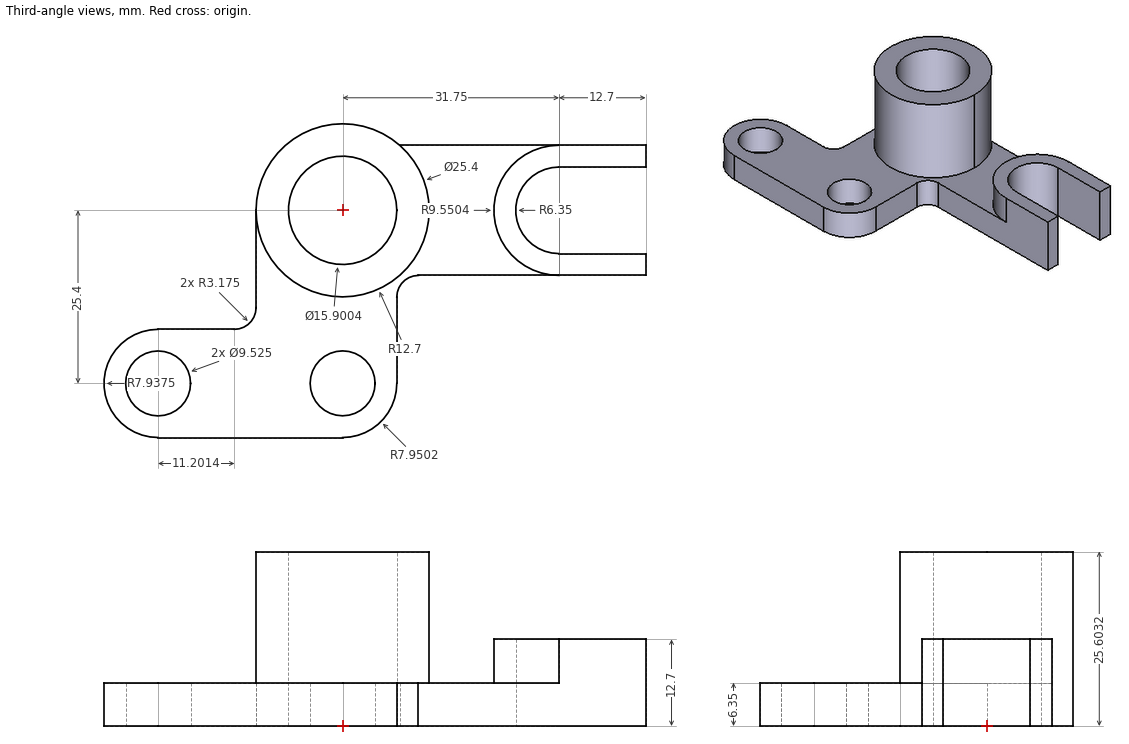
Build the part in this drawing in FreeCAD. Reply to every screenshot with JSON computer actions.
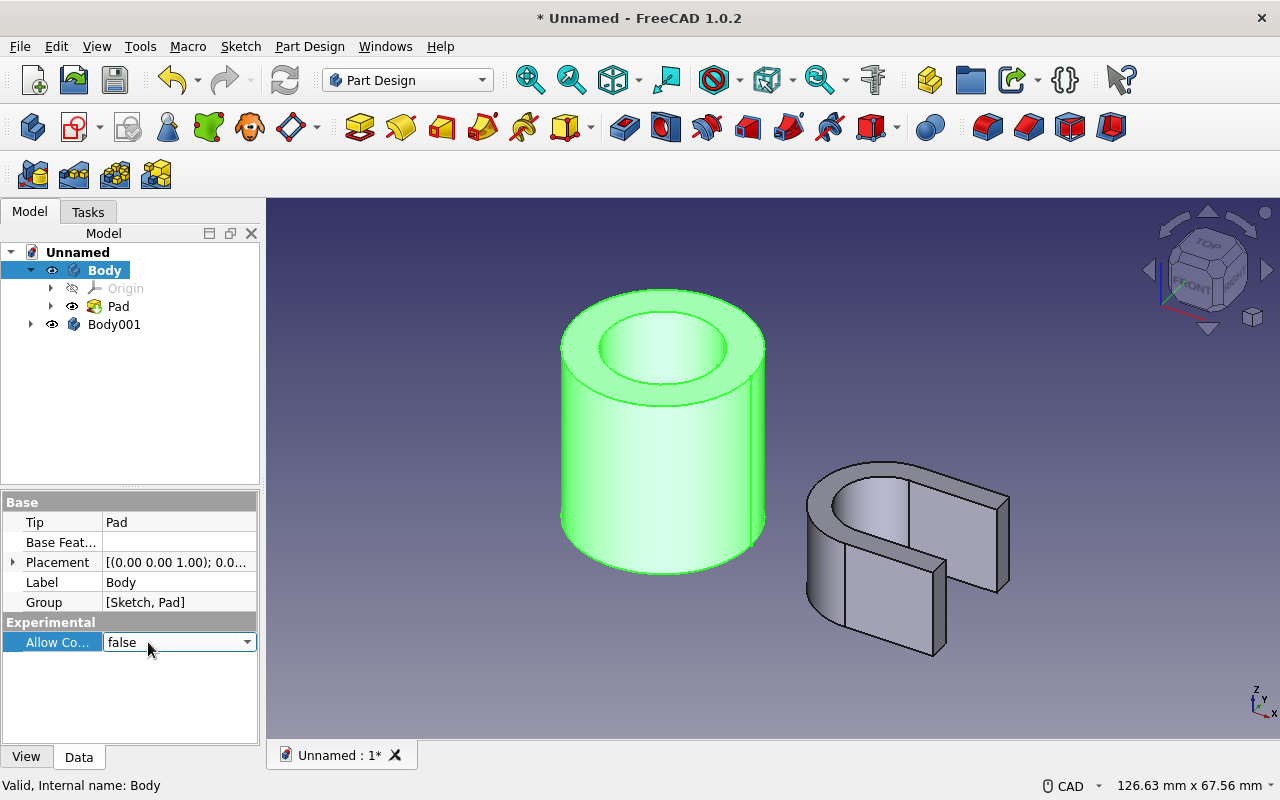
{"action": "left_click", "coordinate": [148, 642]}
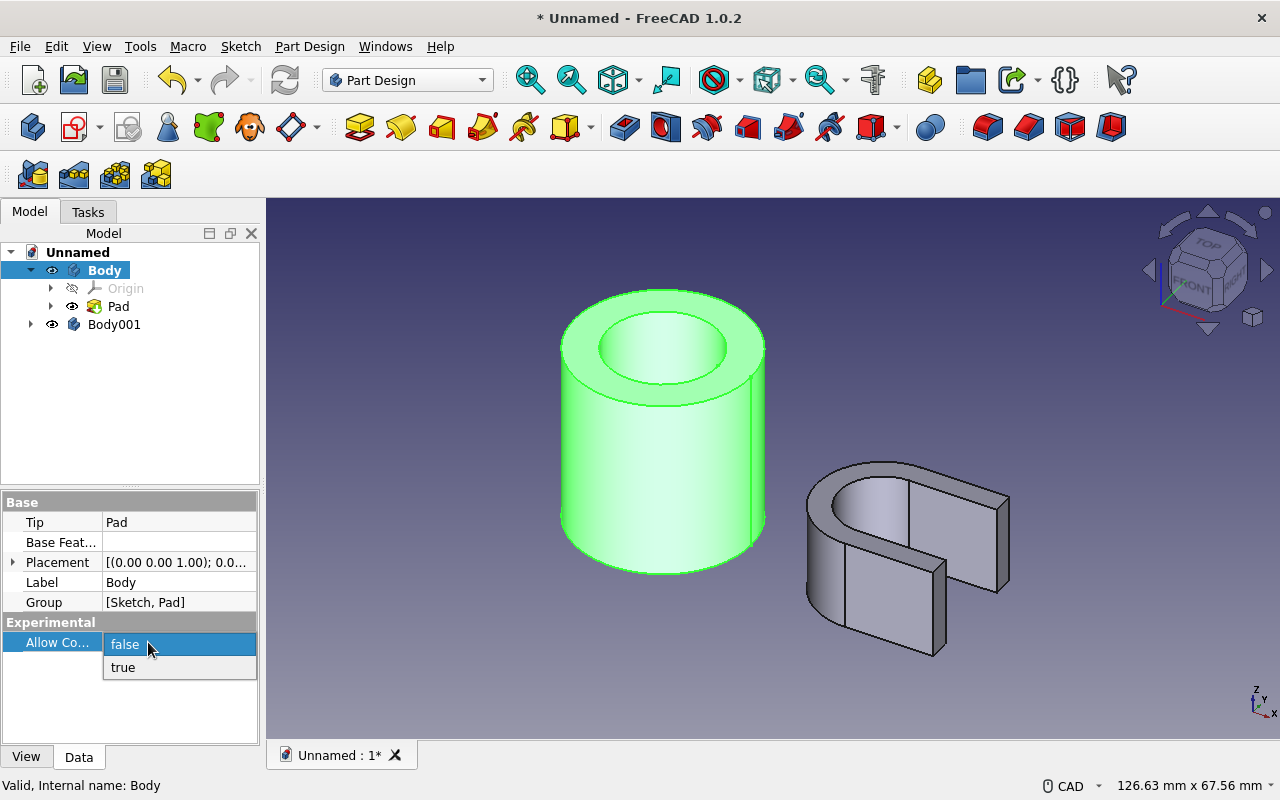
{"action": "left_click", "coordinate": [178, 668]}
{"action": "key", "text": "Return"}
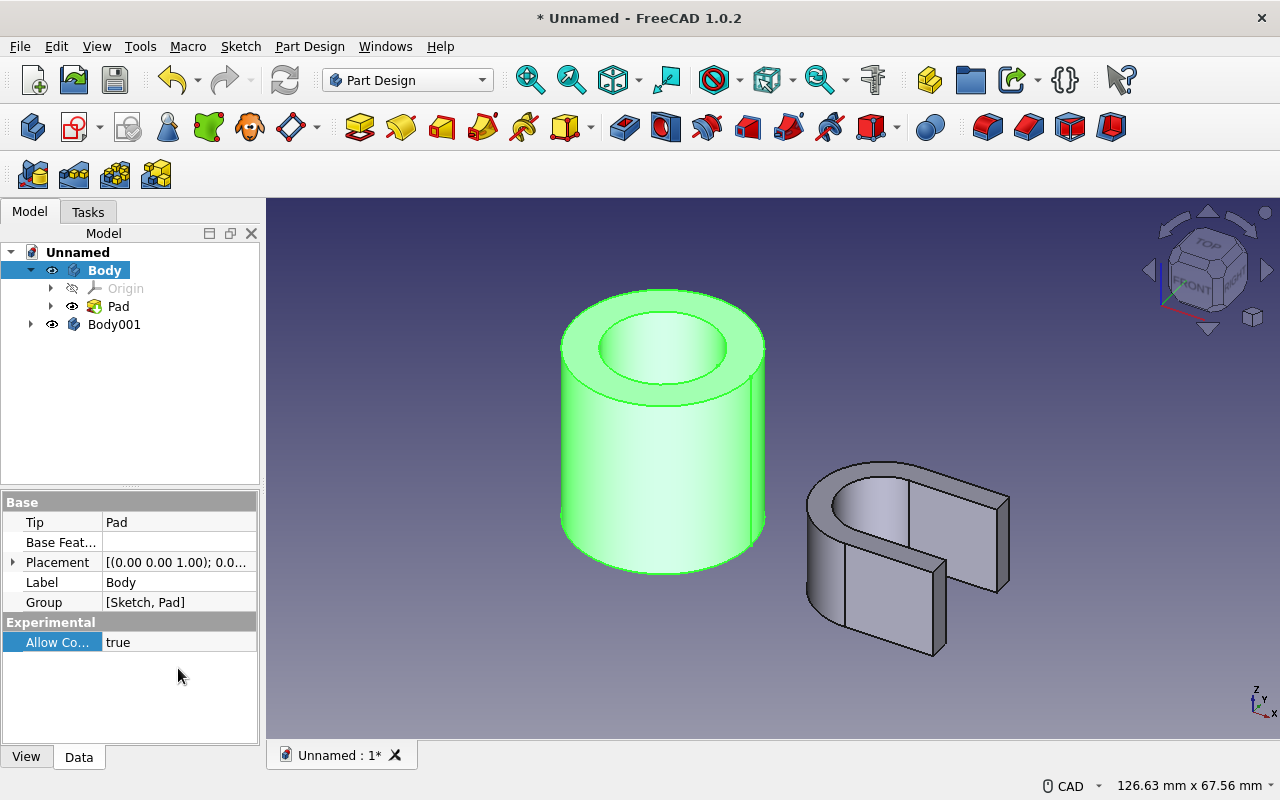
{"action": "left_click", "coordinate": [97, 324]}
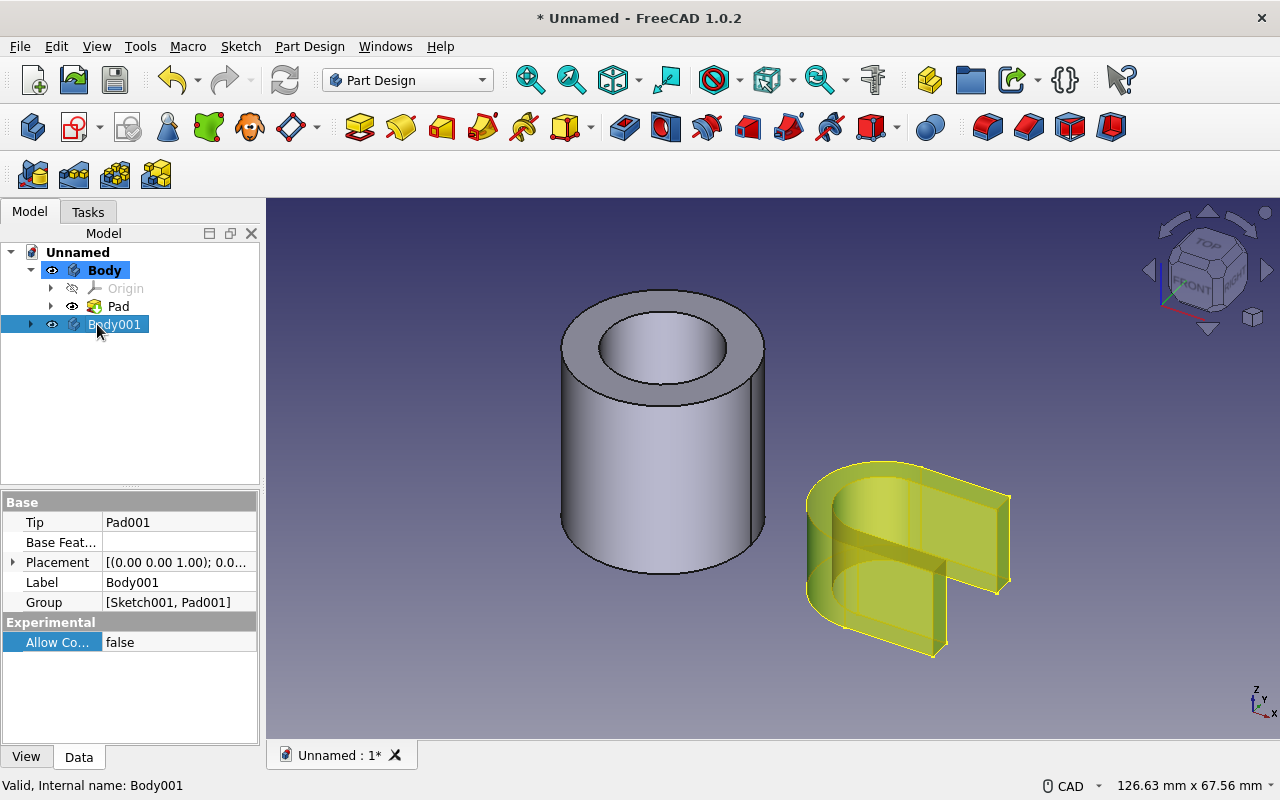
{"action": "left_click", "coordinate": [931, 128]}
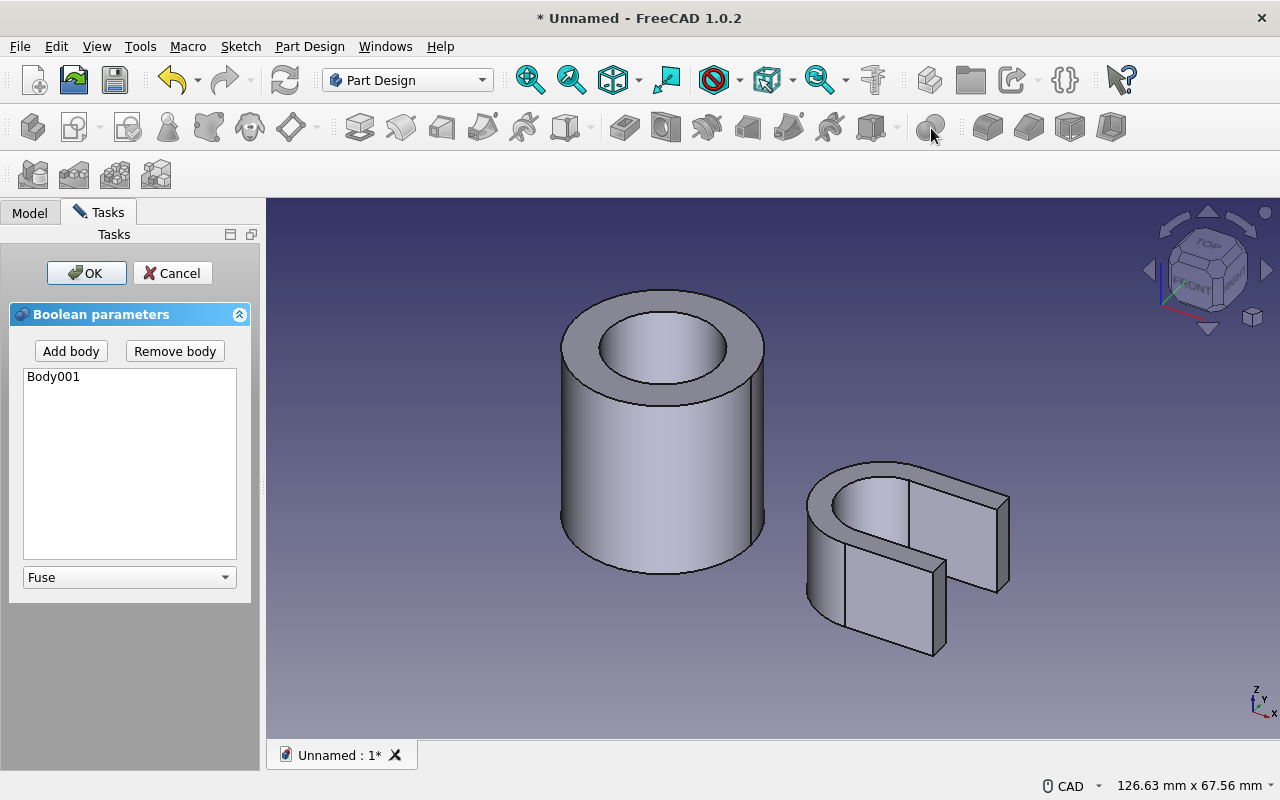
{"action": "left_click", "coordinate": [87, 273]}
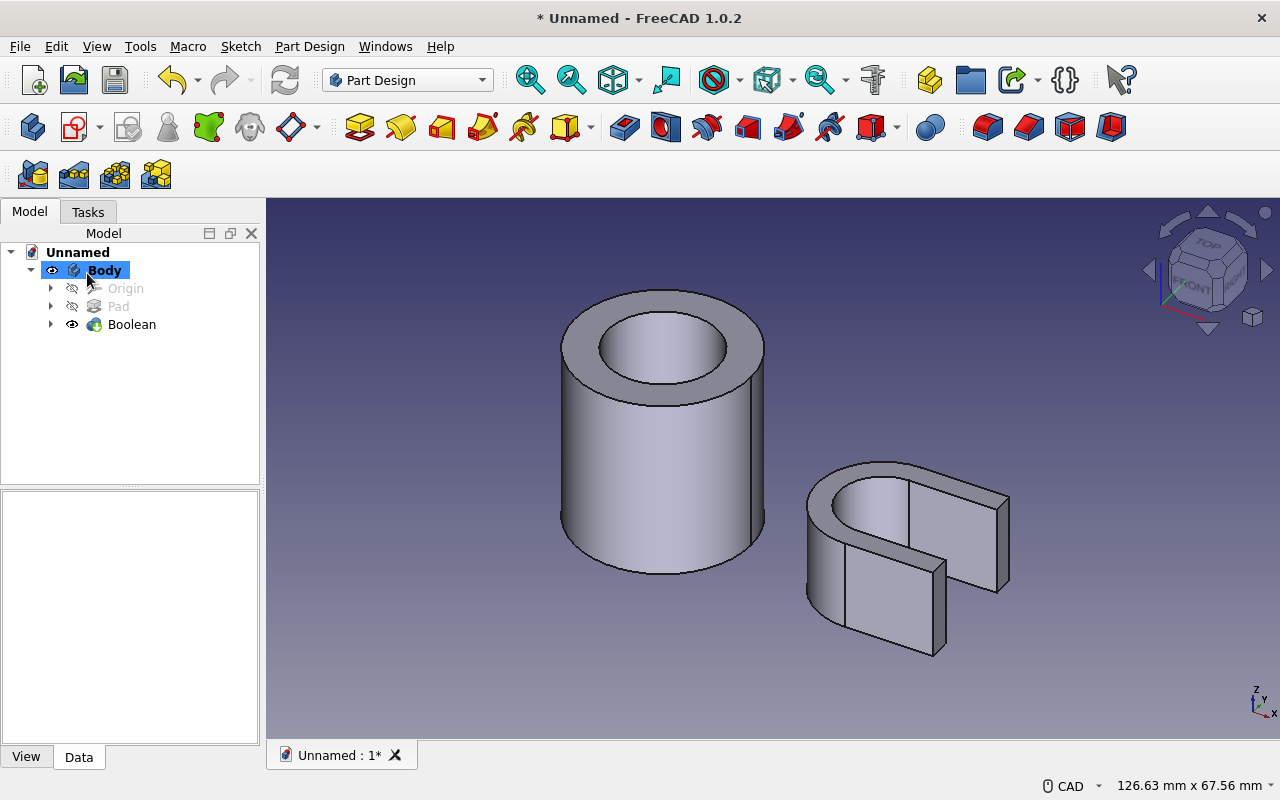
{"action": "left_click", "coordinate": [74, 128]}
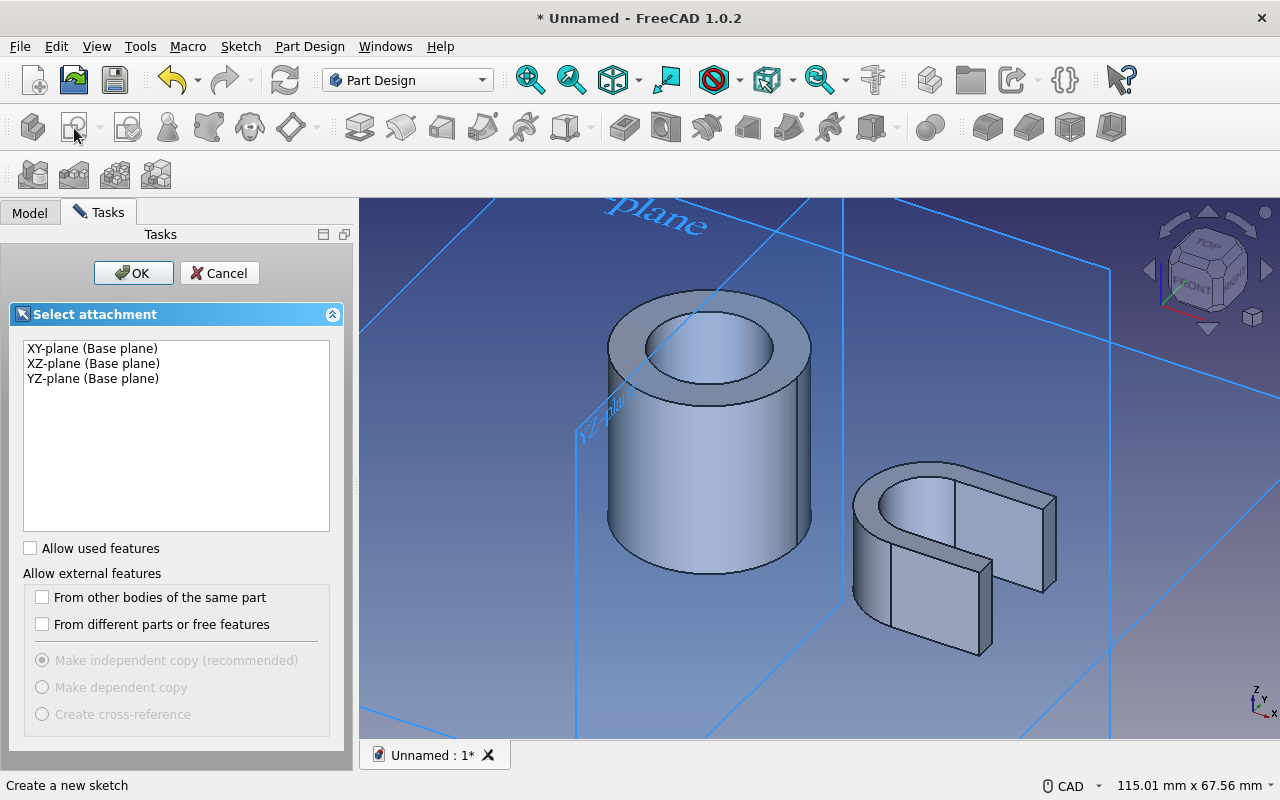
{"action": "left_click", "coordinate": [84, 348]}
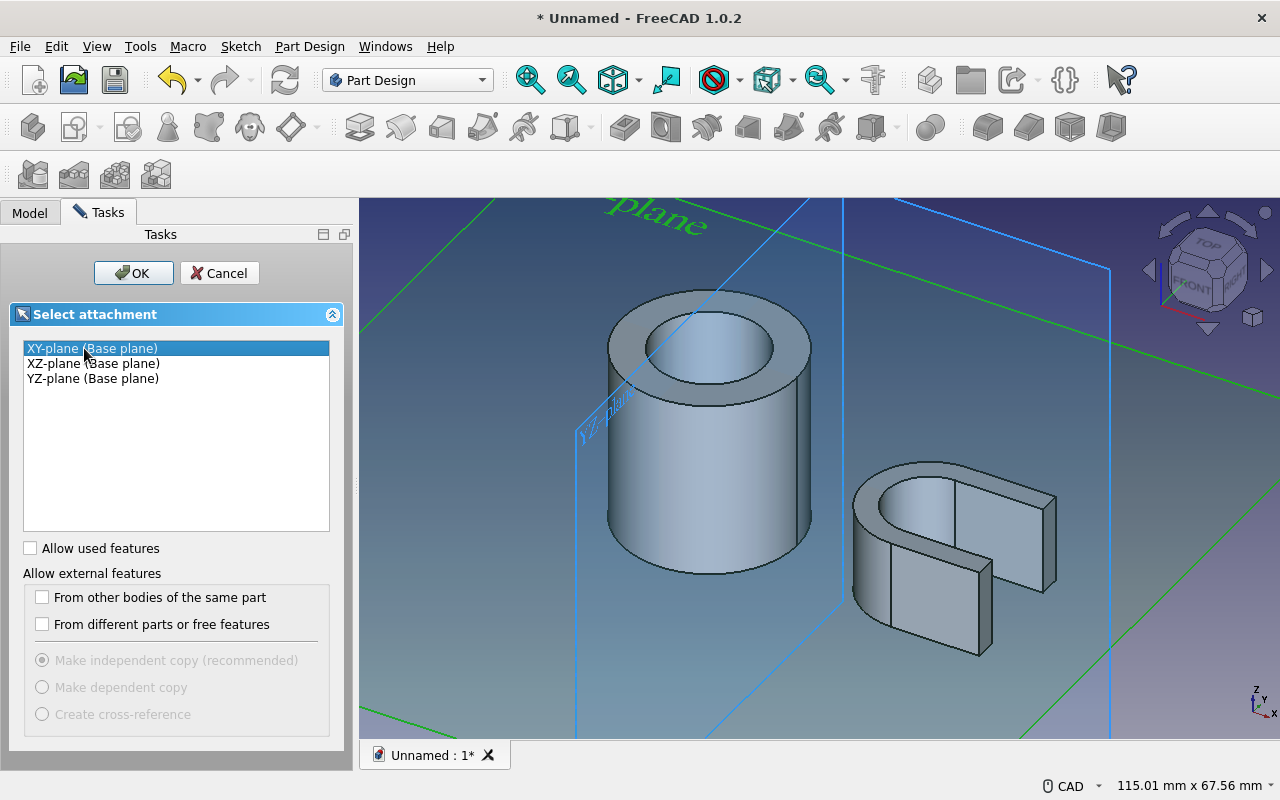
{"action": "left_click", "coordinate": [134, 273]}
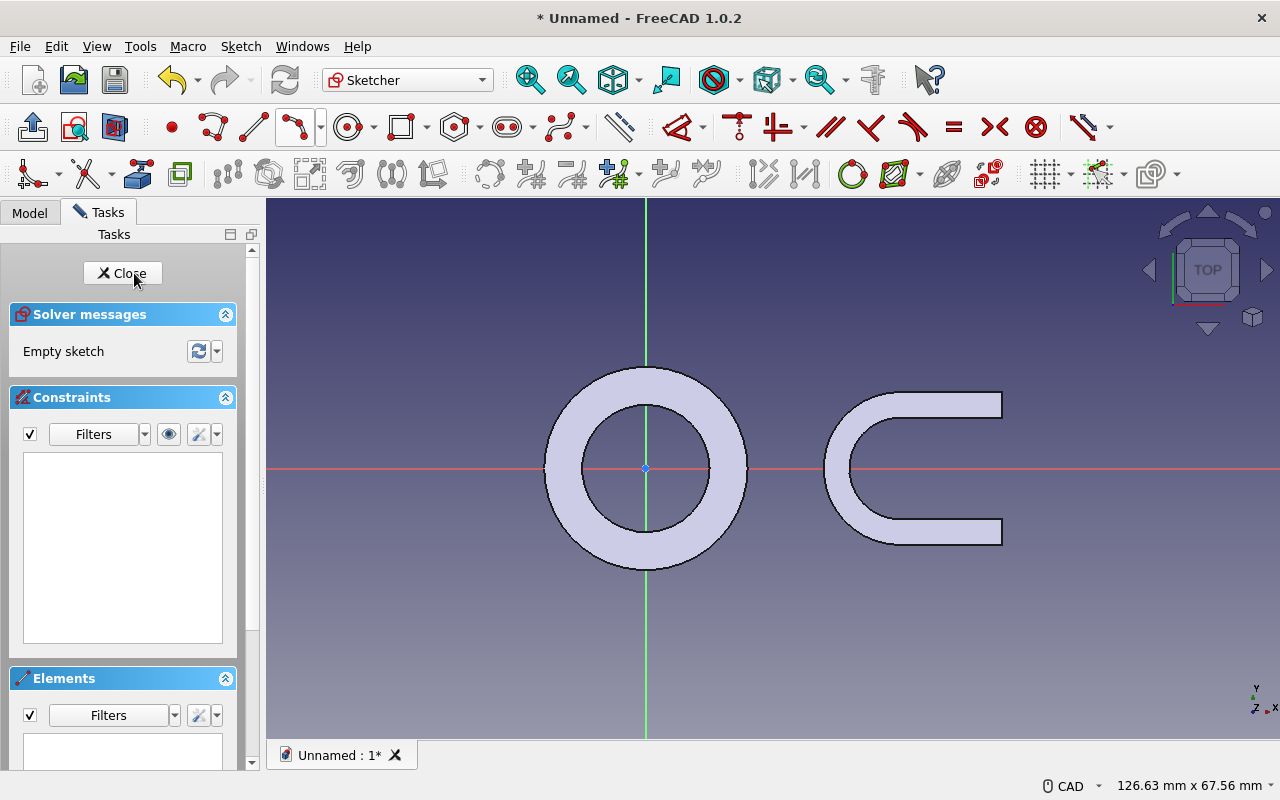
{"action": "left_click", "coordinate": [115, 128]}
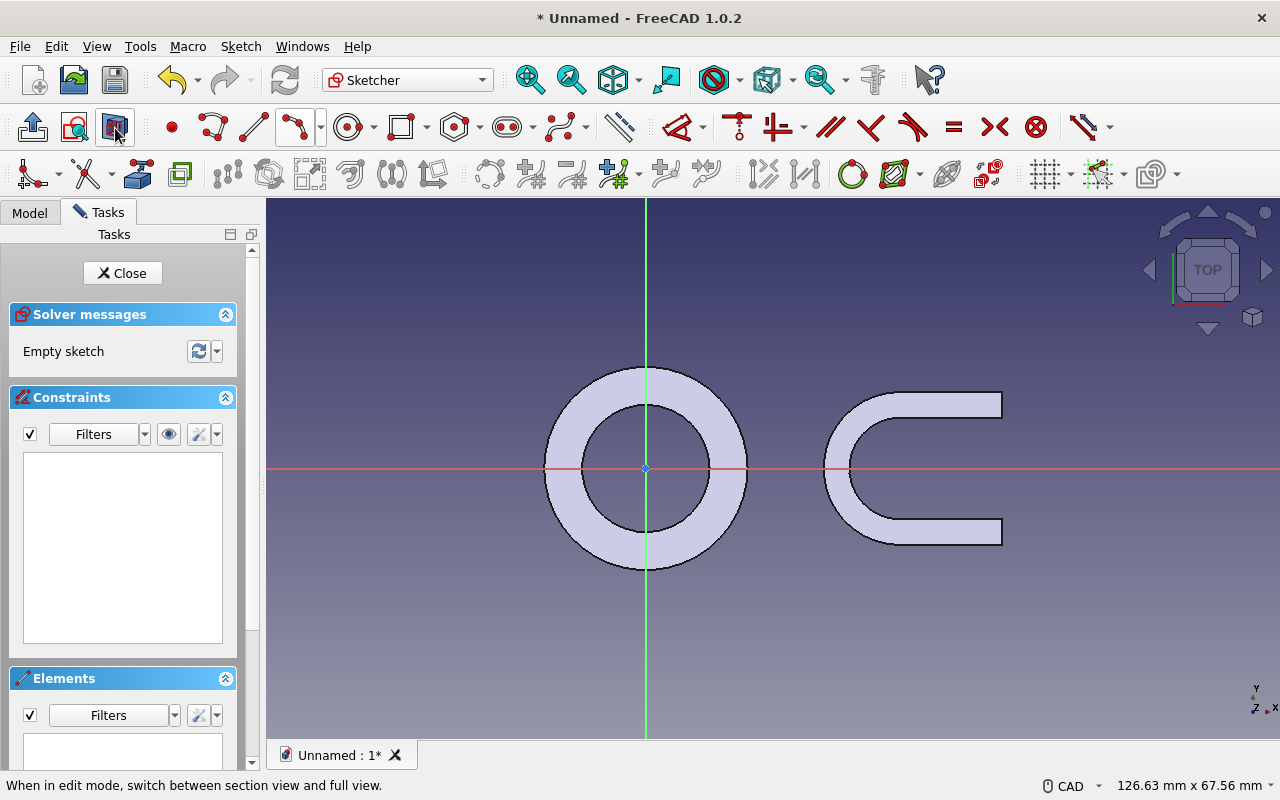
{"action": "scroll", "coordinate": [1028, 226], "scroll_direction": "down", "scroll_amount": 1}